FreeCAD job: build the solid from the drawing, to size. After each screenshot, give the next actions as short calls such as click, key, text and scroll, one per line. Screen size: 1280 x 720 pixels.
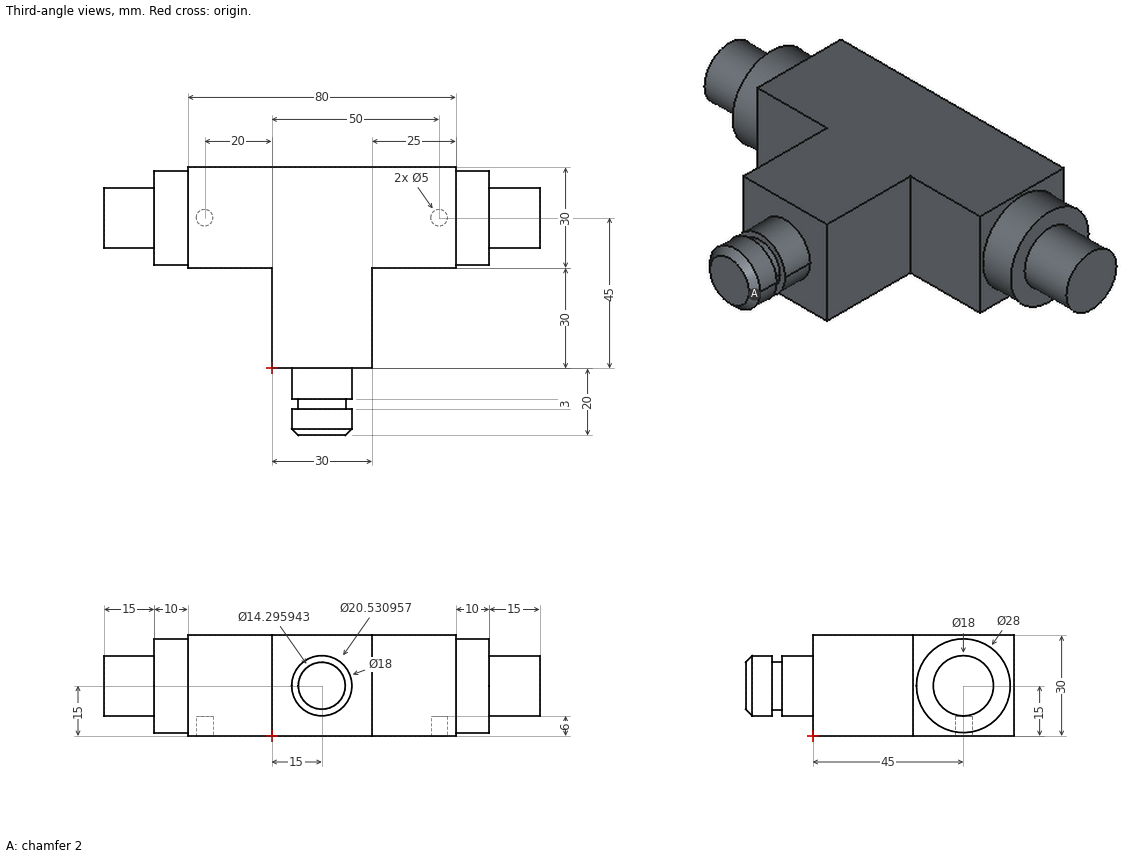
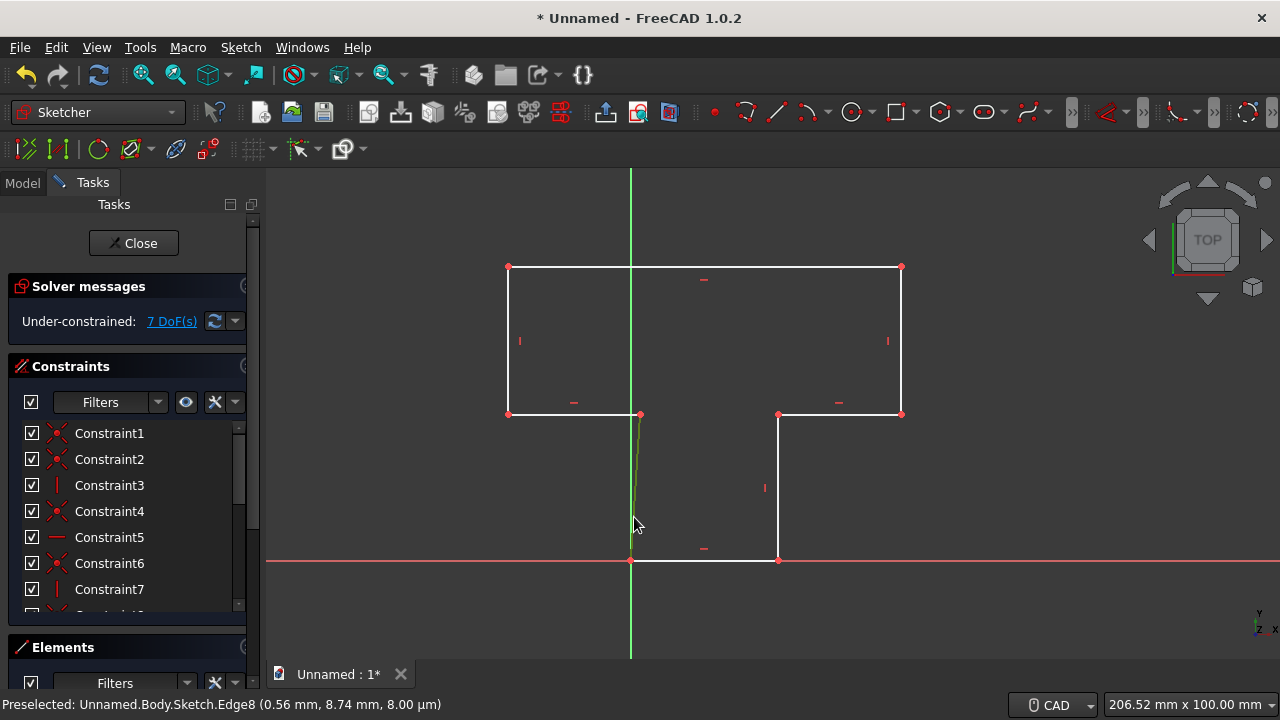
key(v)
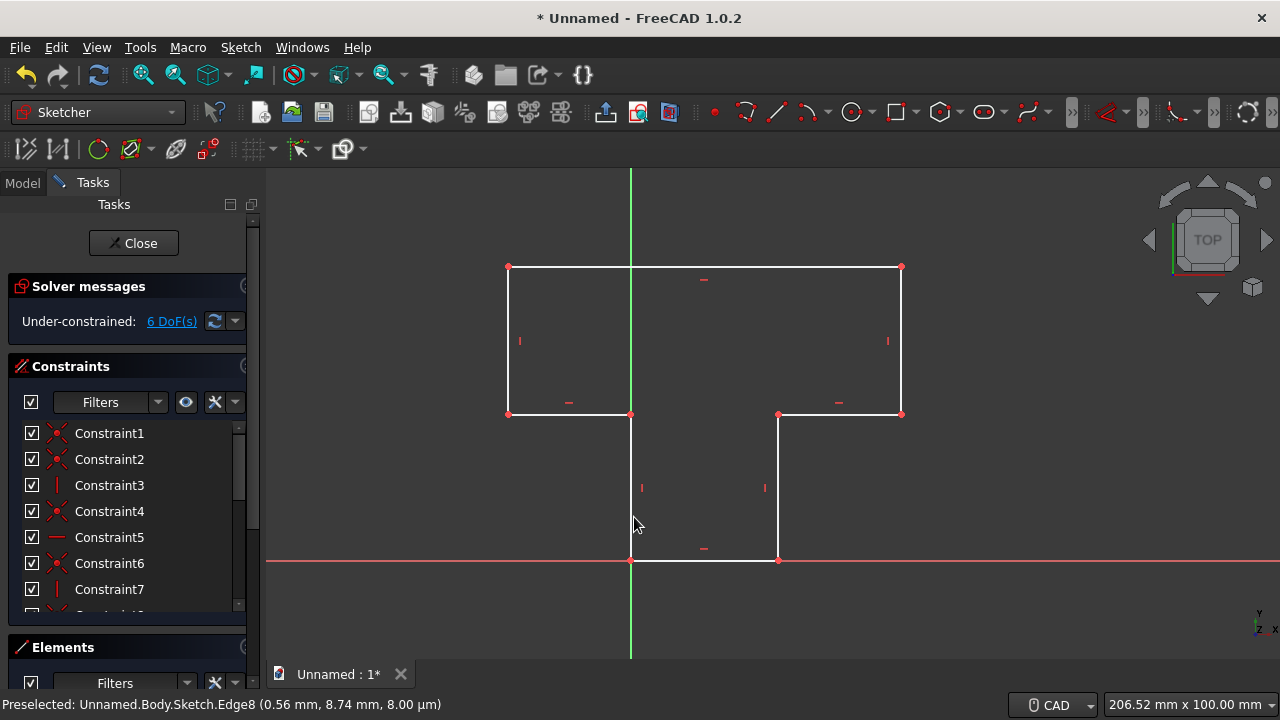
key(d)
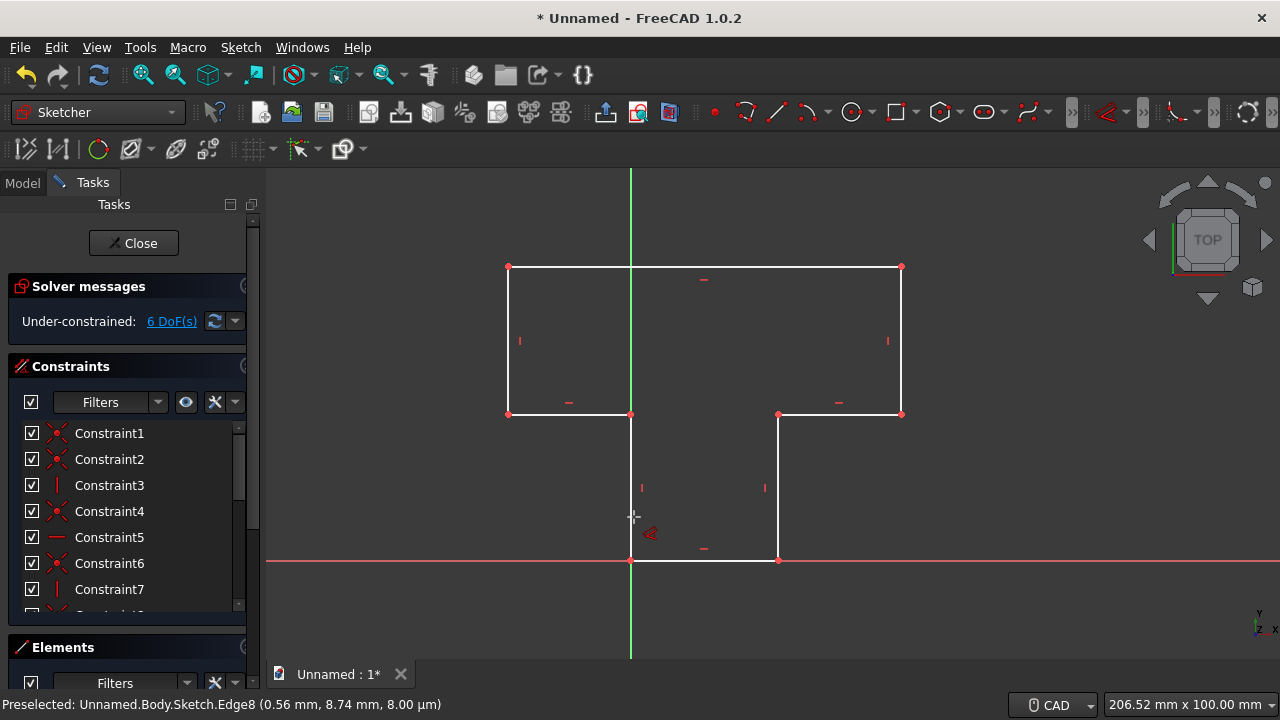
click(675, 561)
click(704, 595)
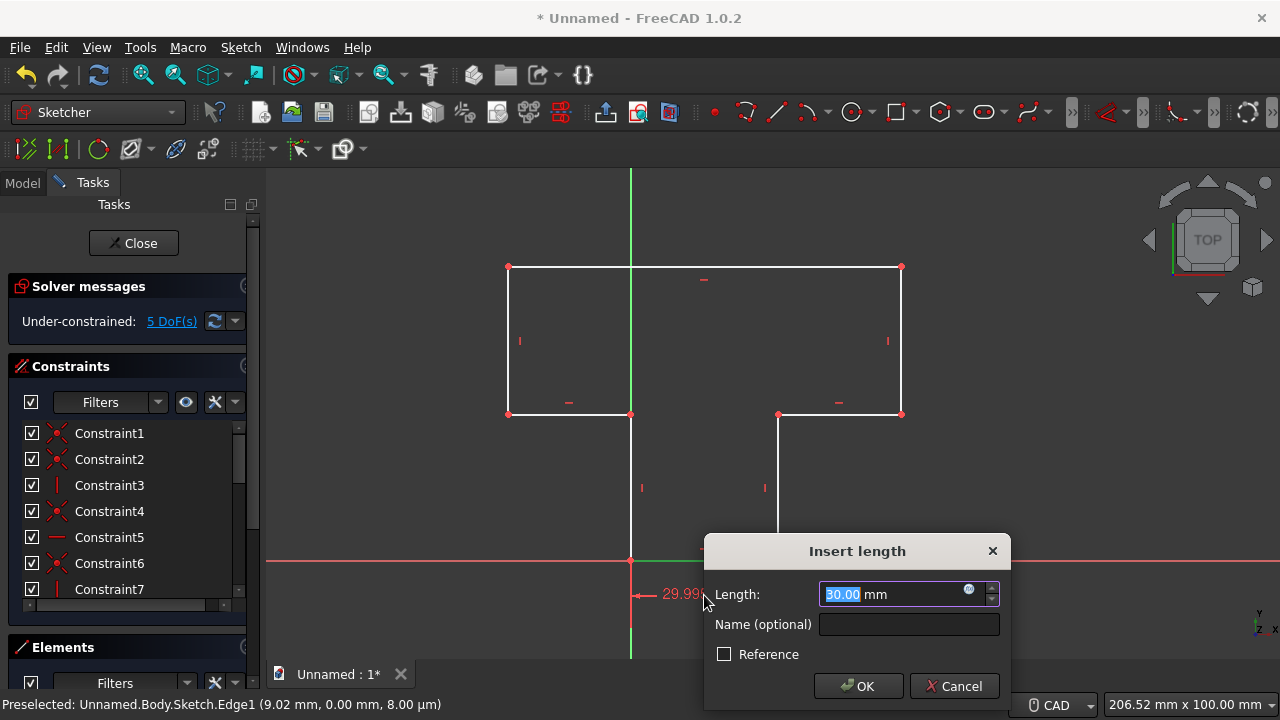
text(30)
key(Return)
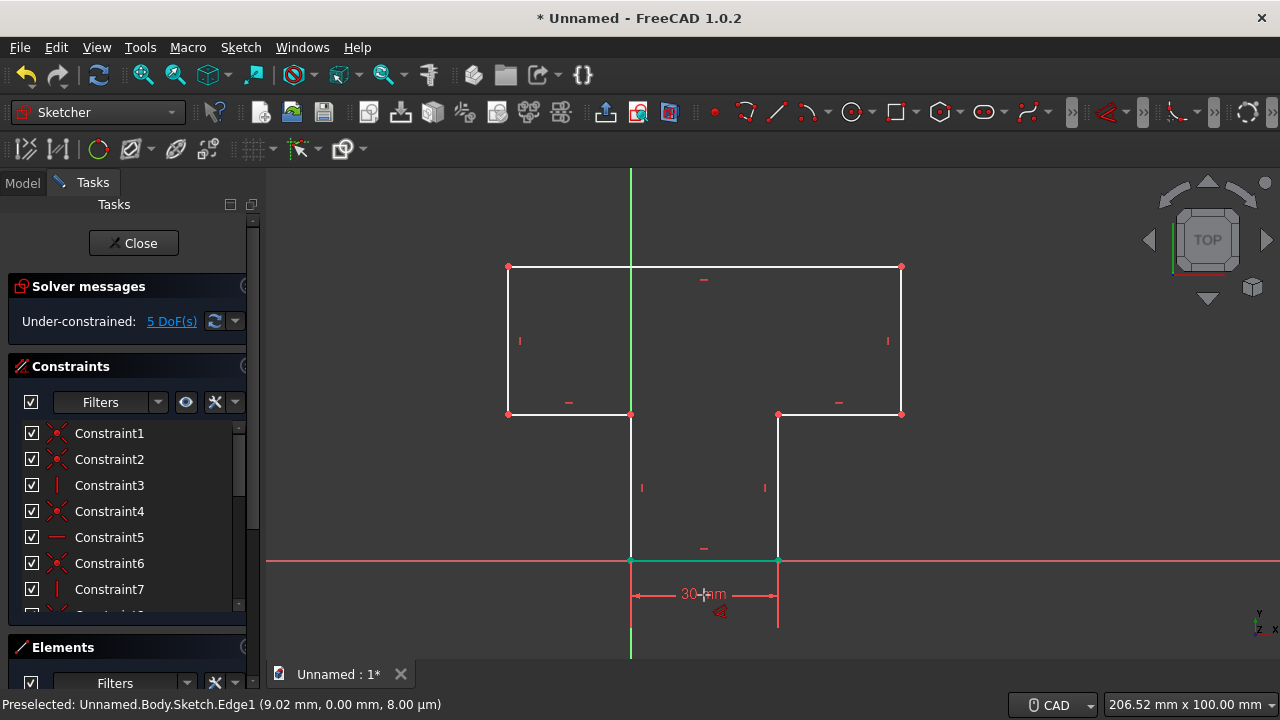
click(778, 517)
click(812, 488)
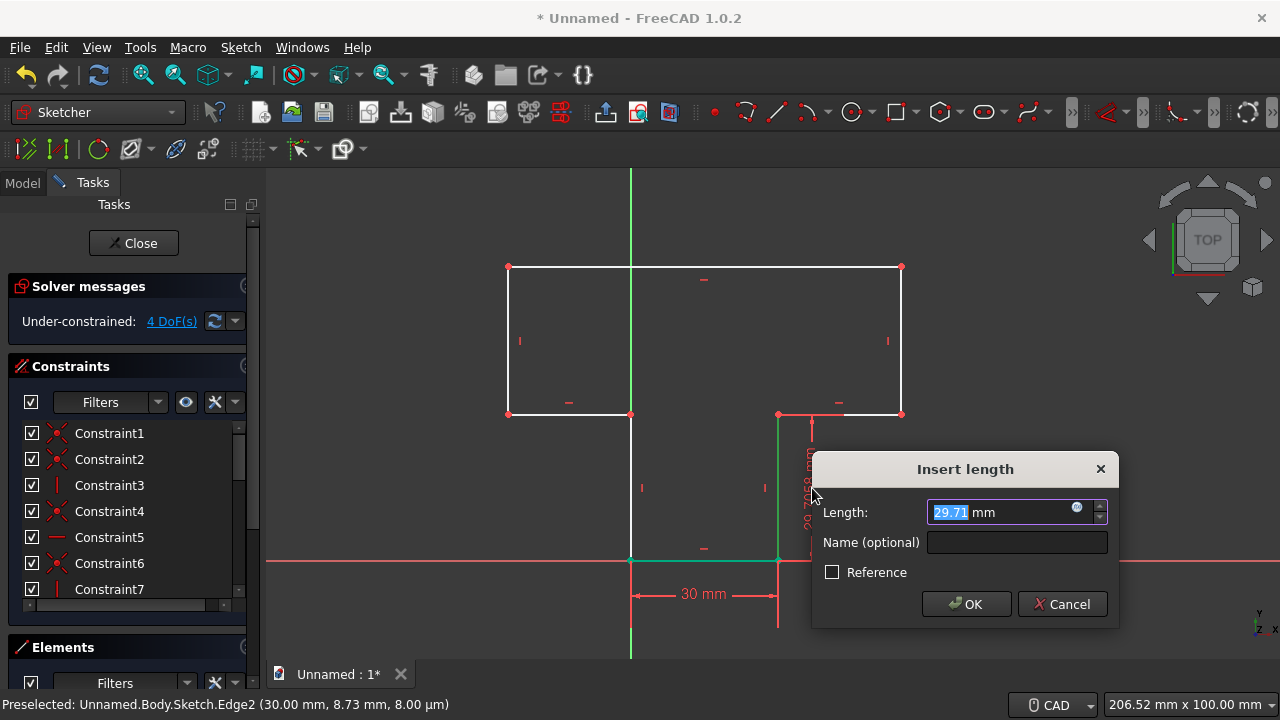
text(30)
key(Return)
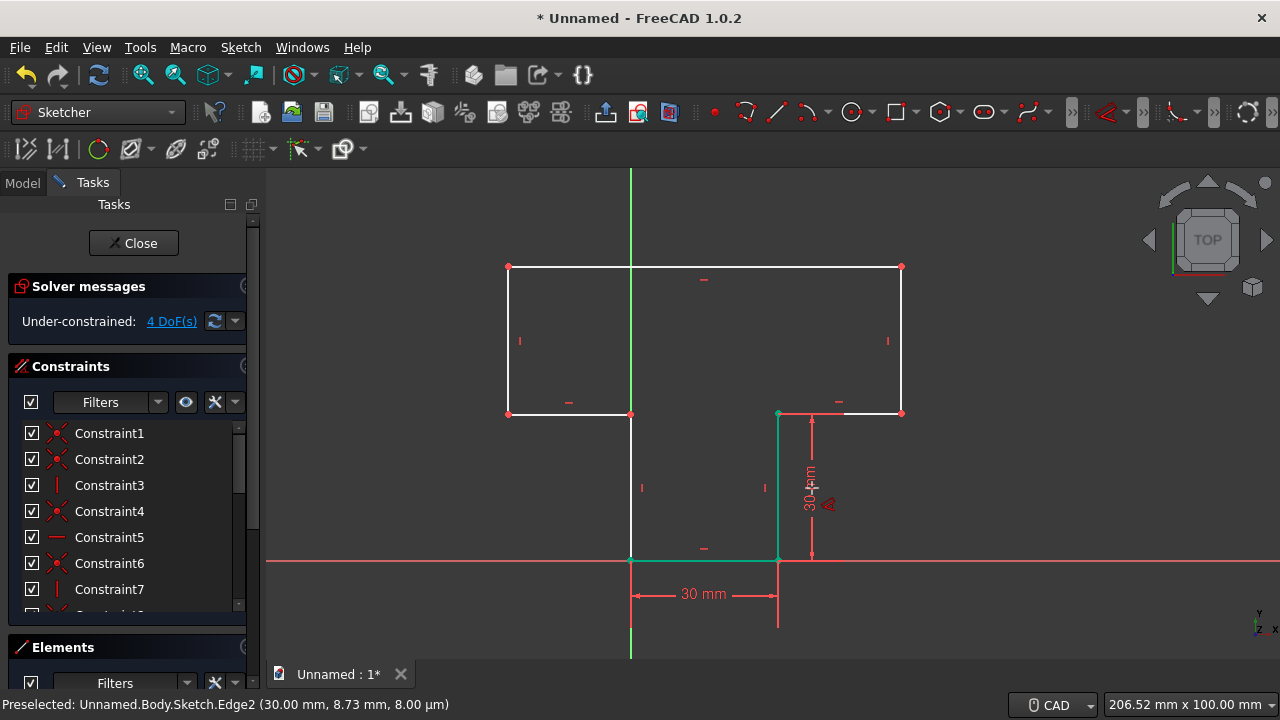
click(815, 414)
click(840, 448)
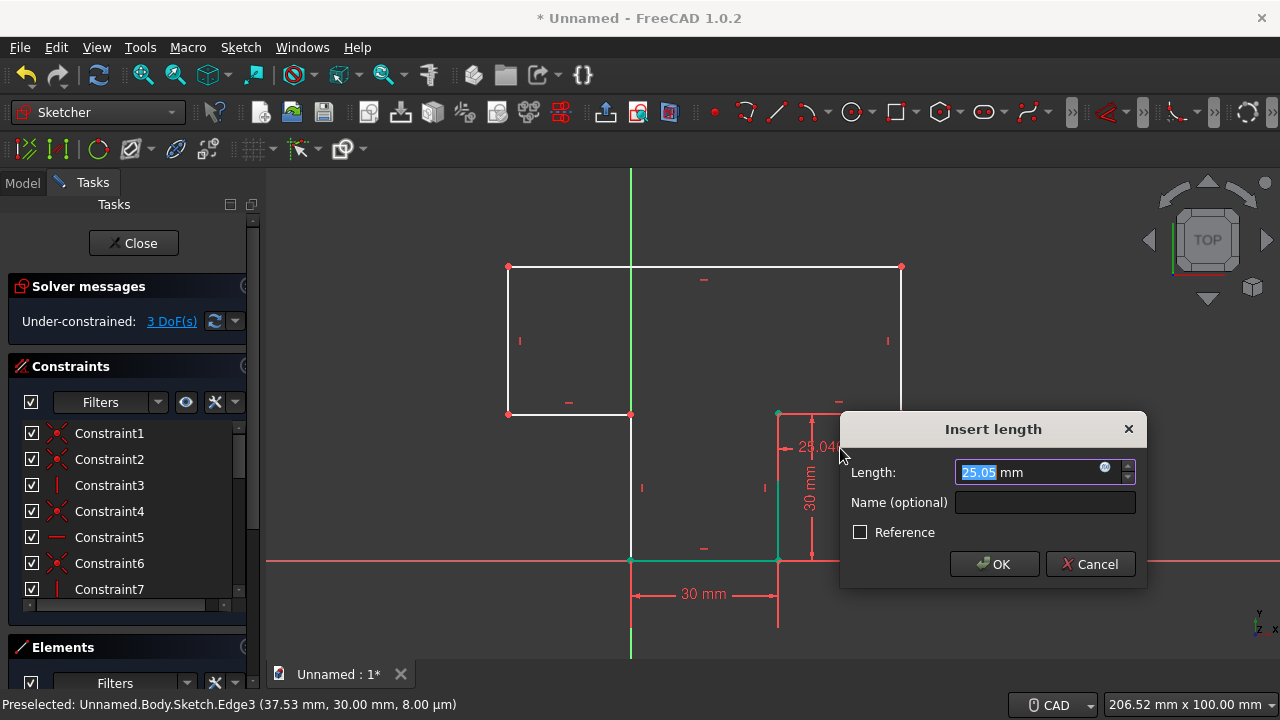
text(25)
key(Return)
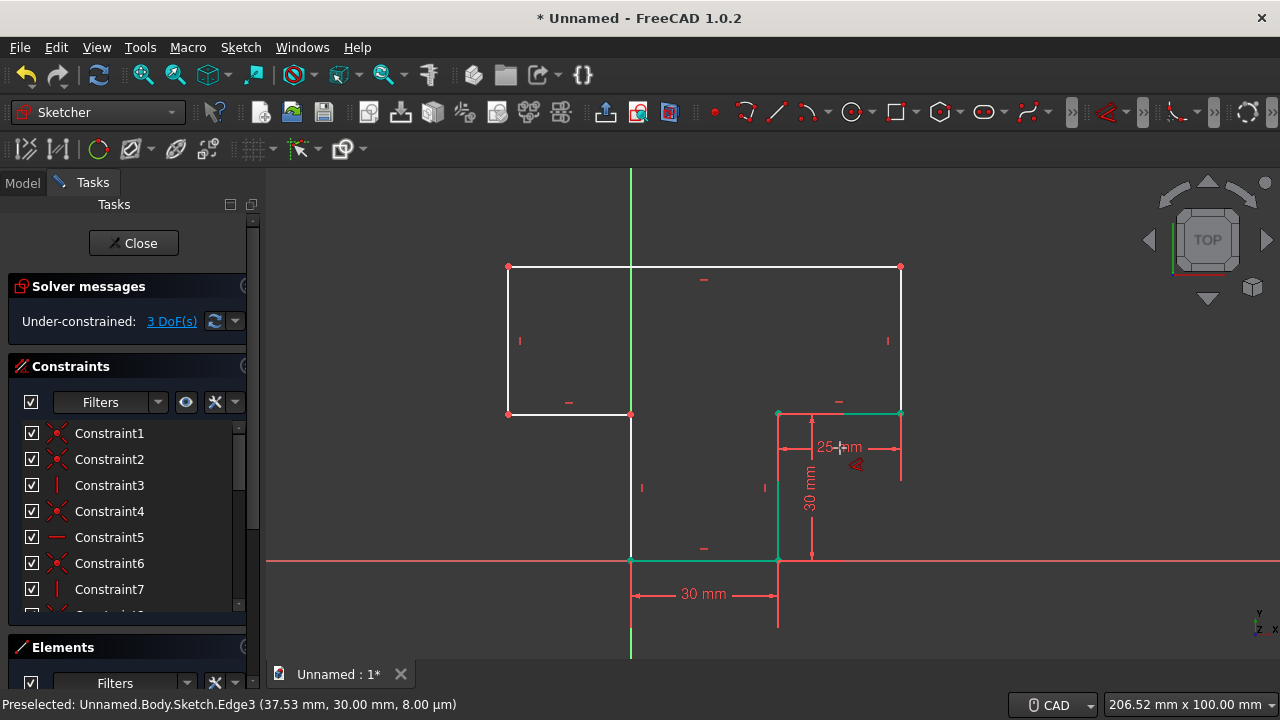
click(901, 370)
click(935, 340)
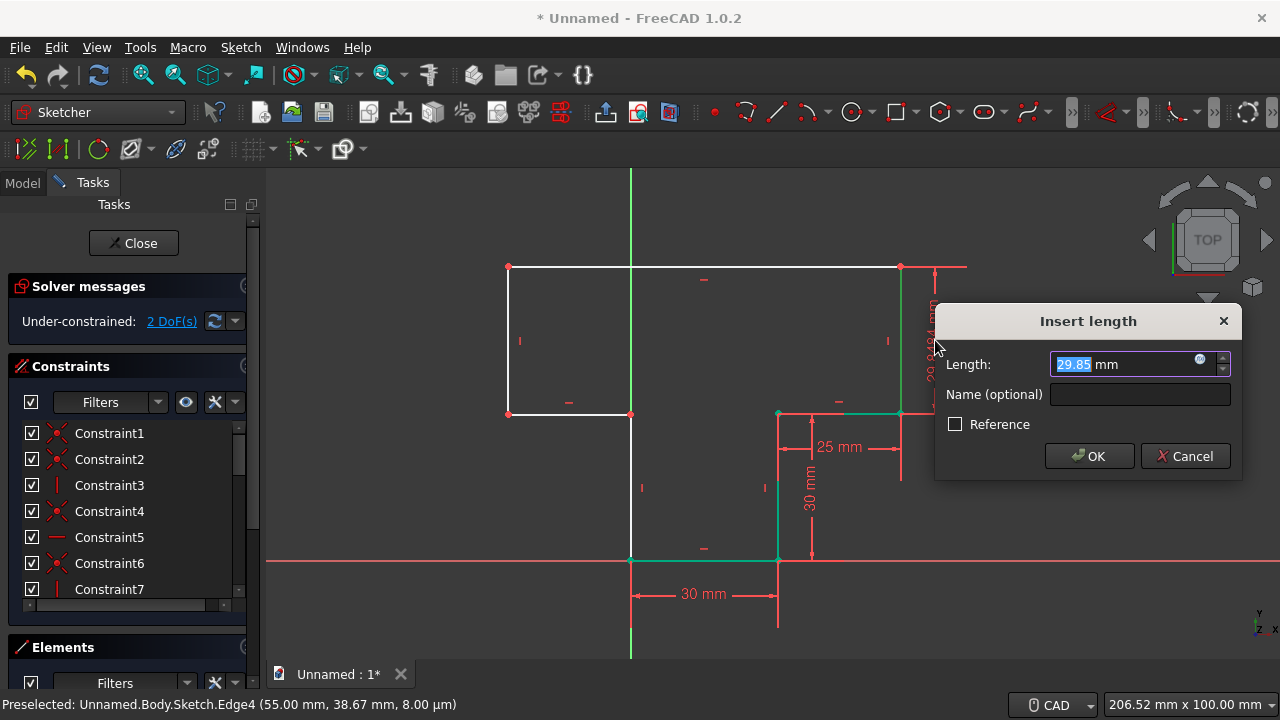
text(30)
key(Return)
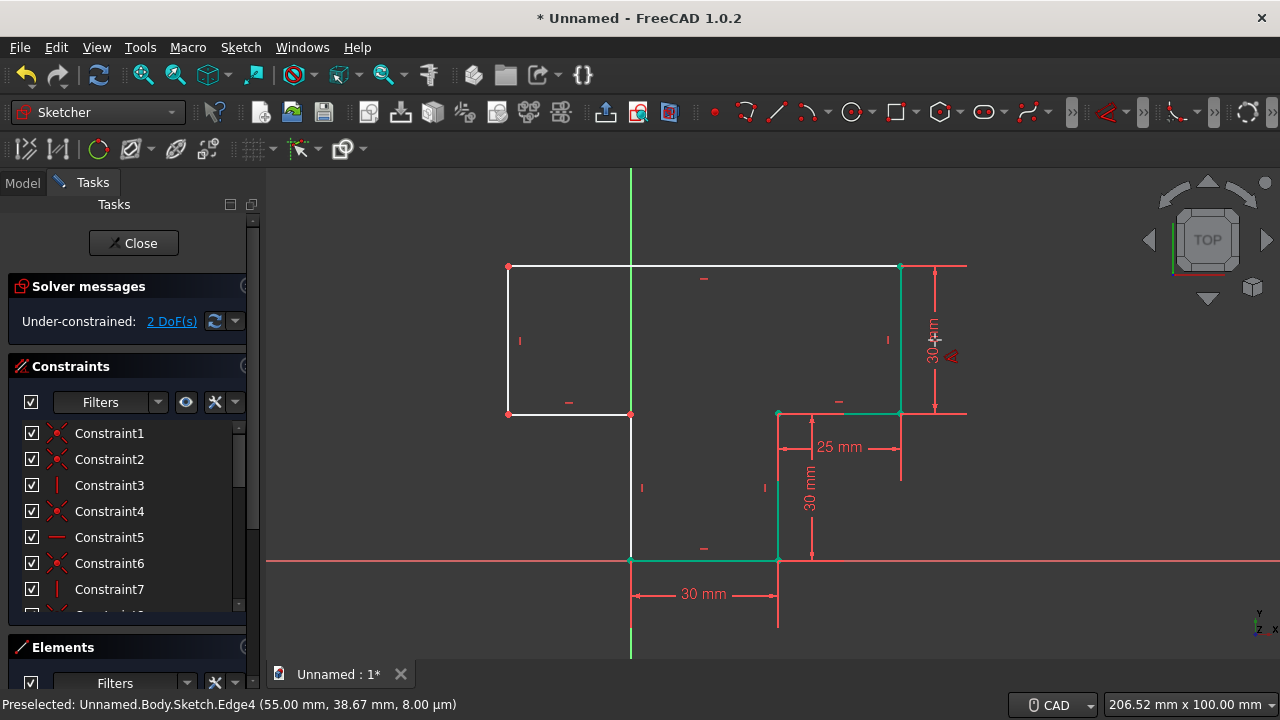
click(783, 266)
click(704, 232)